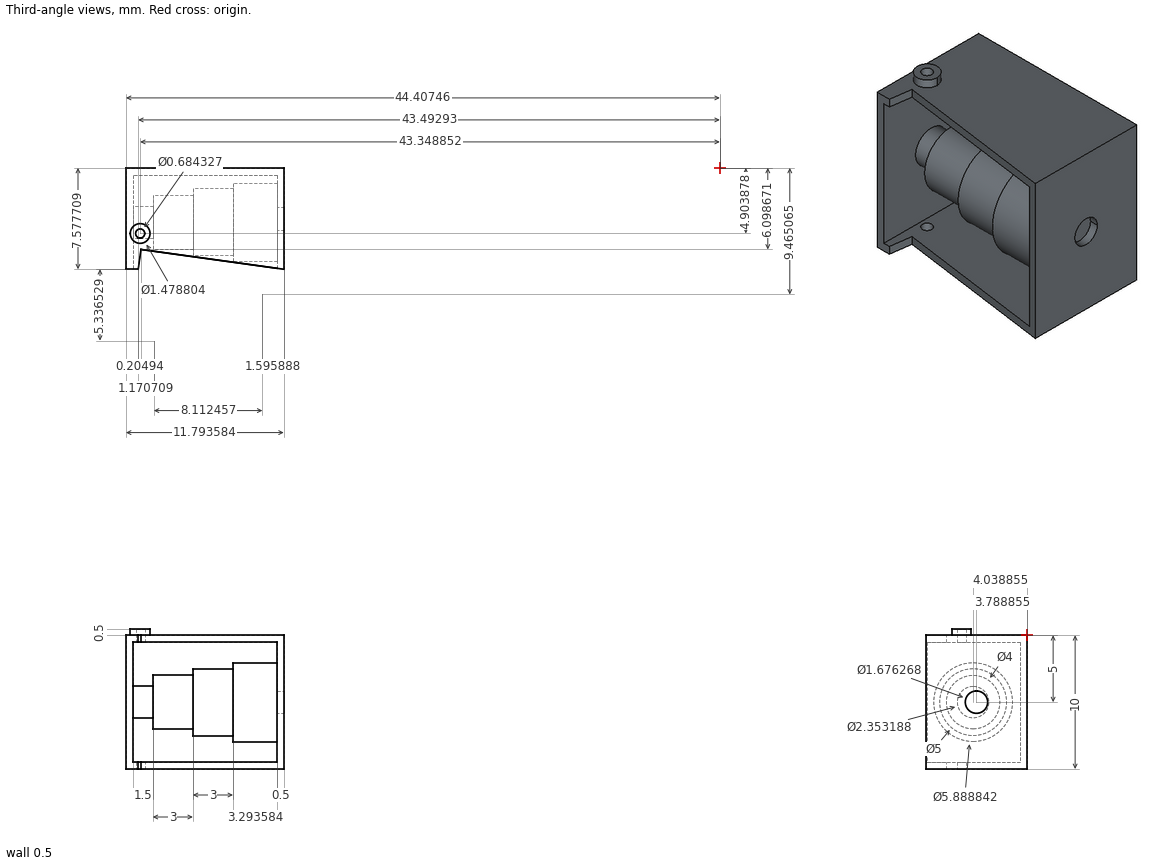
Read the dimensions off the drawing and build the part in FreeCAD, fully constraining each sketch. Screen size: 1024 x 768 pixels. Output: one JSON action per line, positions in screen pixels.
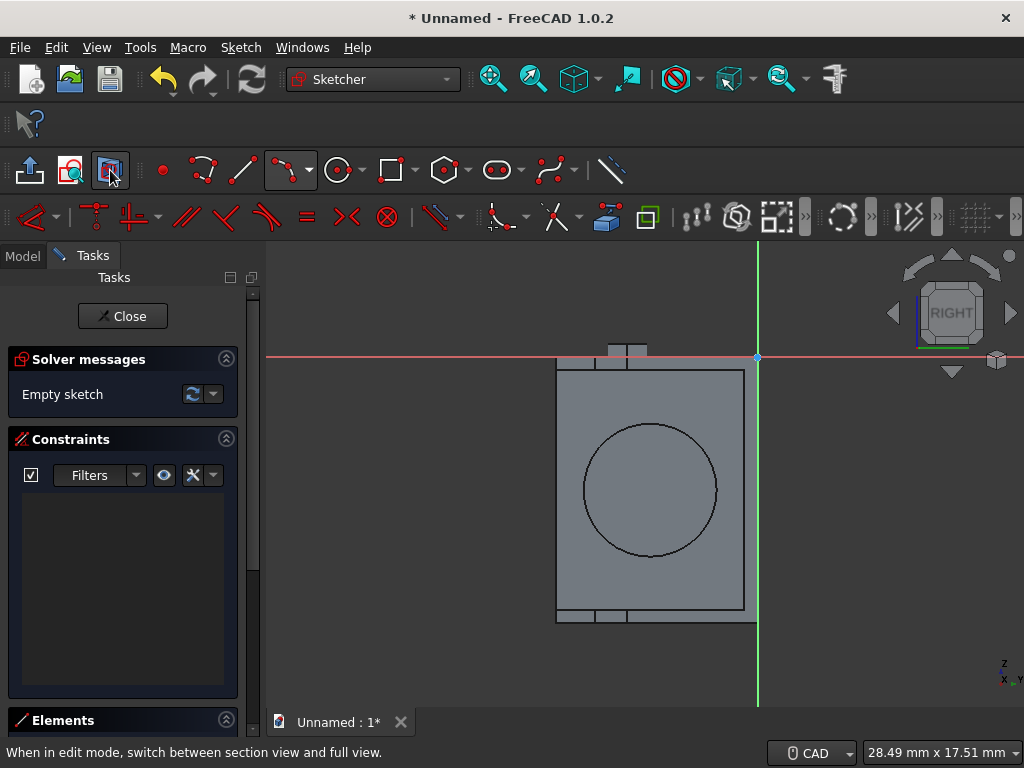
{"action": "scroll", "coordinate": [844, 440], "scroll_direction": "up", "scroll_amount": 2}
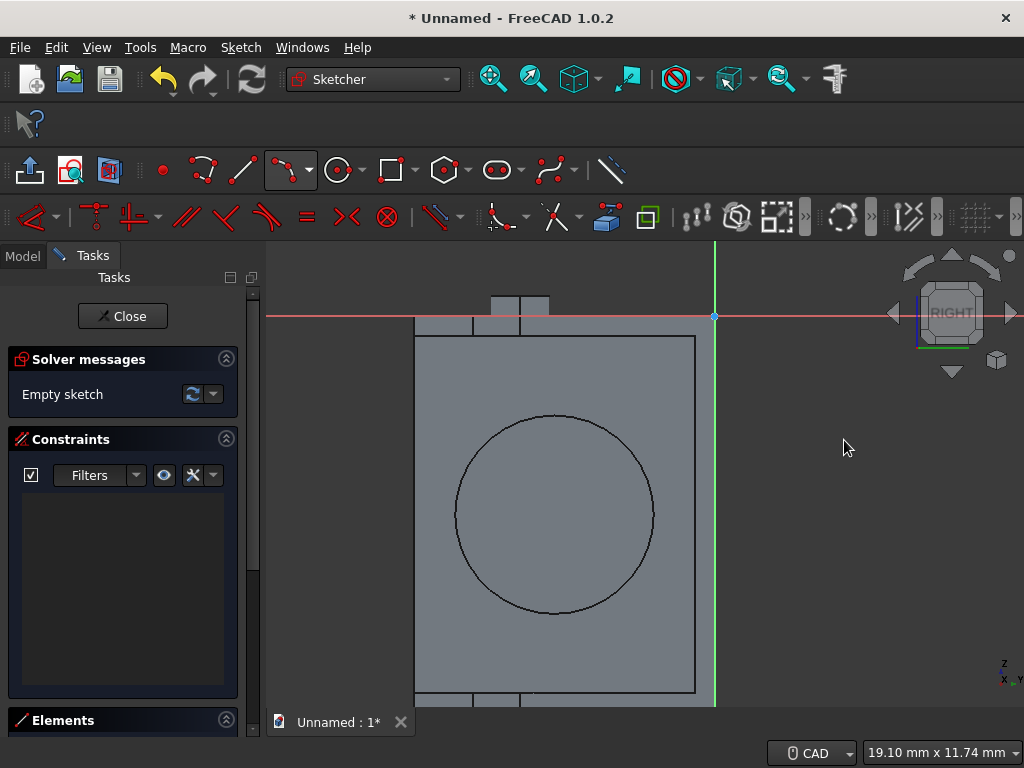
{"action": "left_click", "coordinate": [338, 170]}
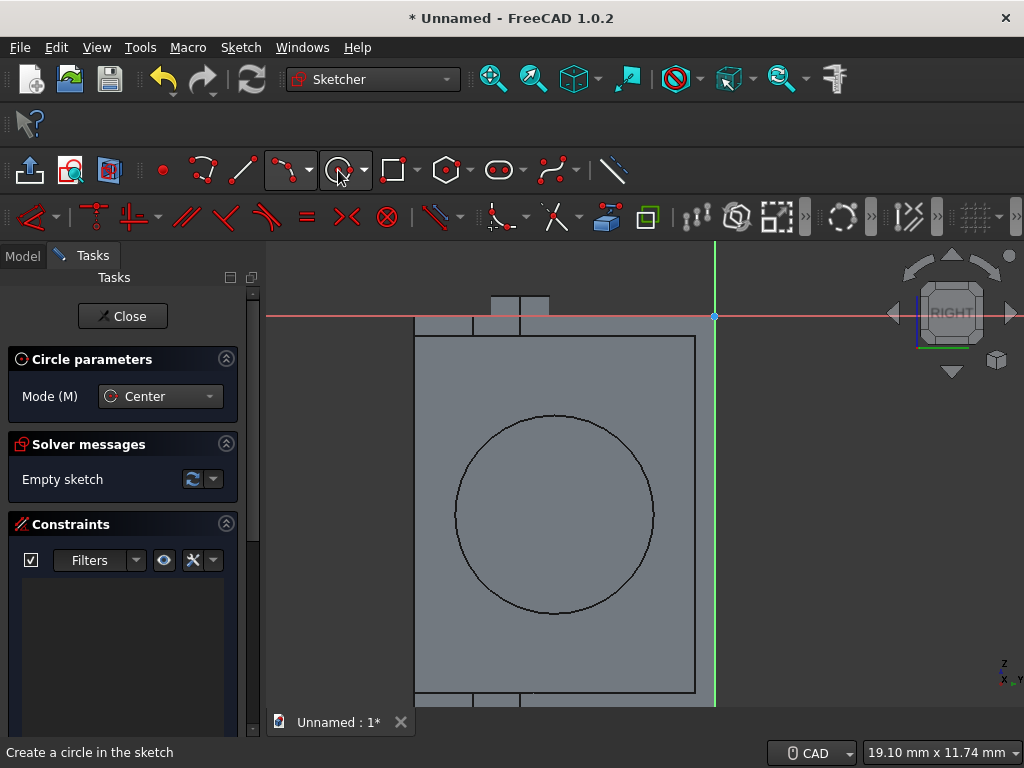
{"action": "left_click", "coordinate": [554, 515]}
{"action": "left_click", "coordinate": [637, 432]}
{"action": "key", "text": "Escape"}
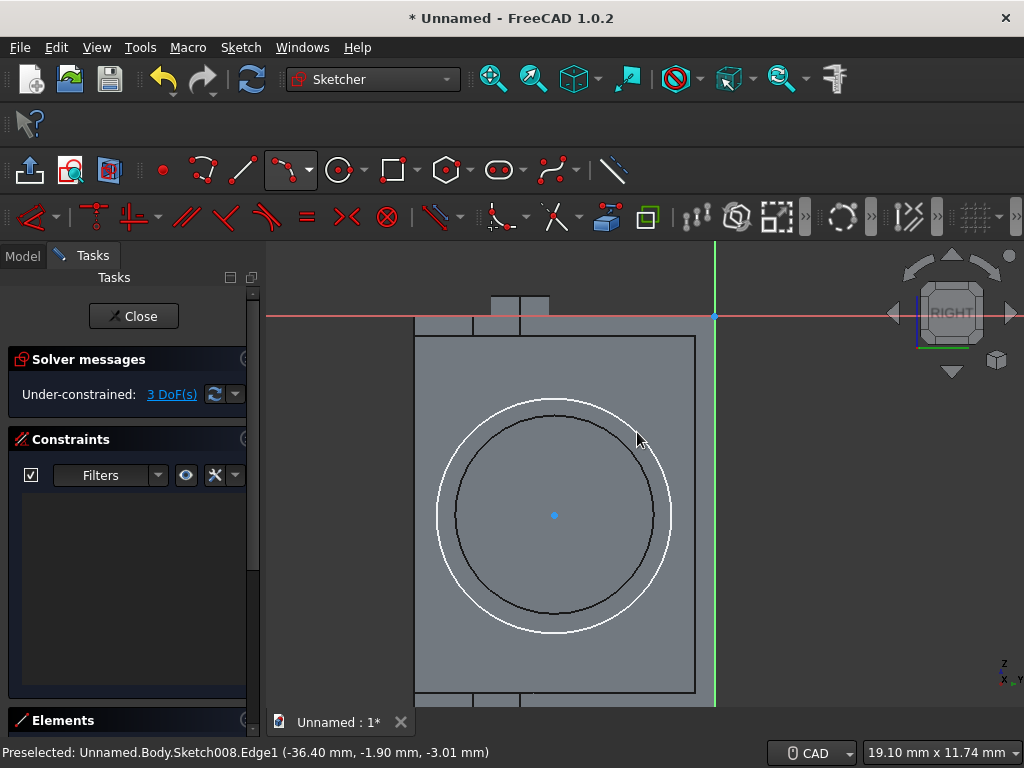
{"action": "left_click", "coordinate": [32, 218]}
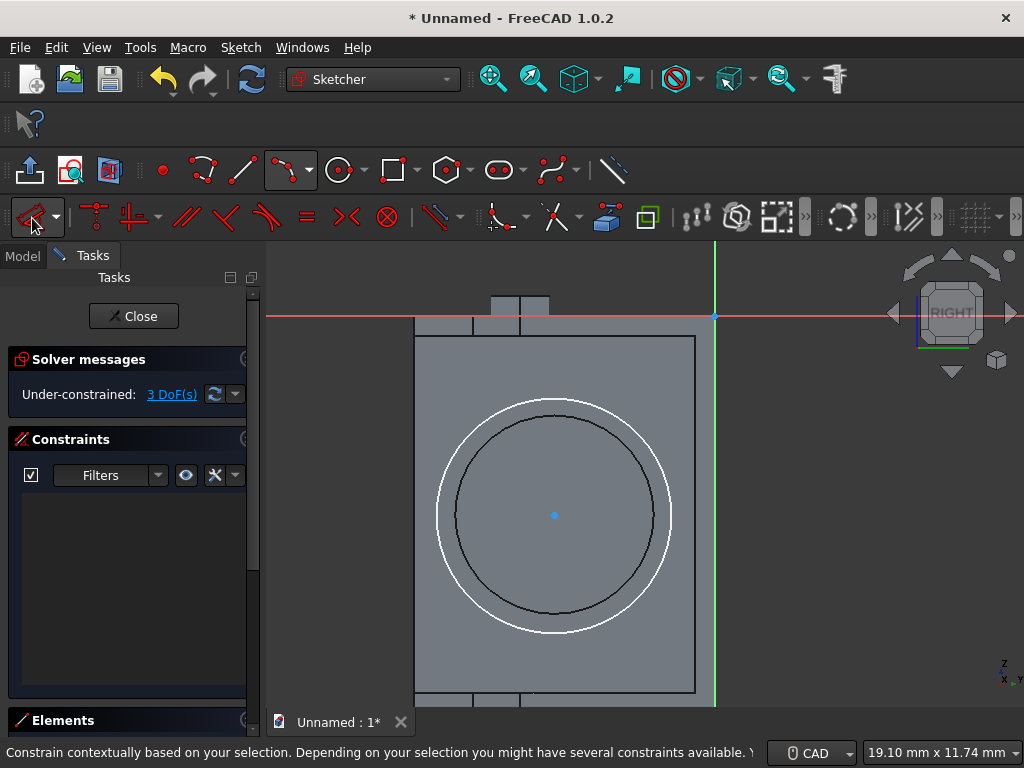
{"action": "left_click", "coordinate": [637, 433]}
{"action": "left_click", "coordinate": [660, 410]}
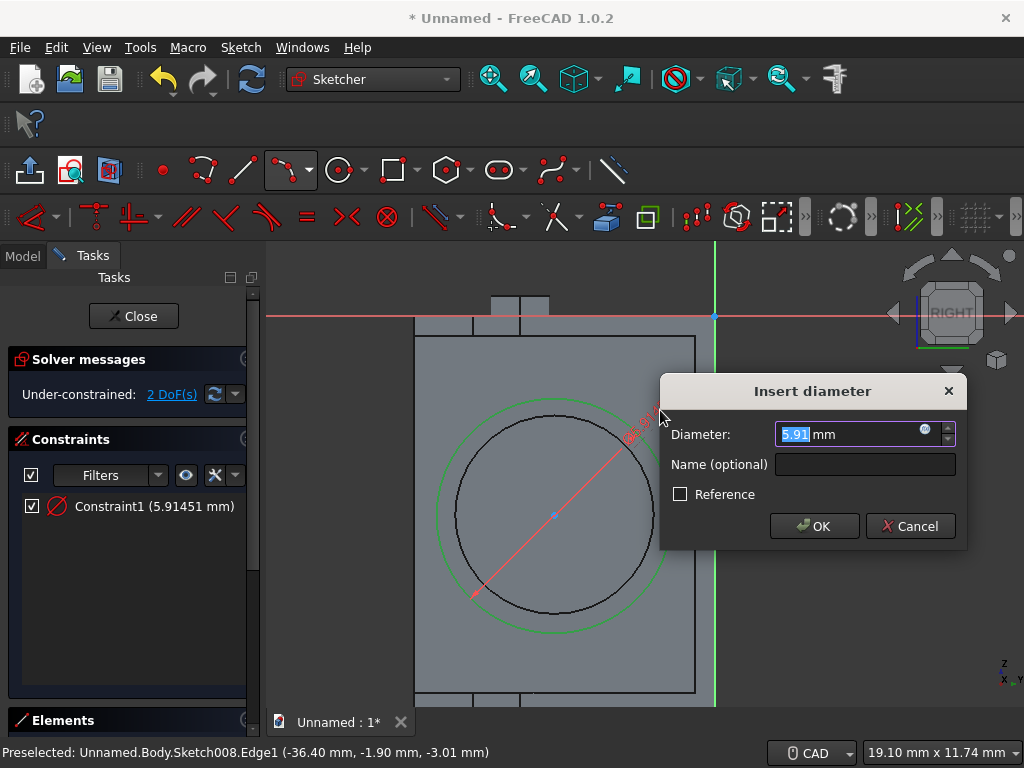
{"action": "type", "text": "5.888842"}
{"action": "key", "text": "Return"}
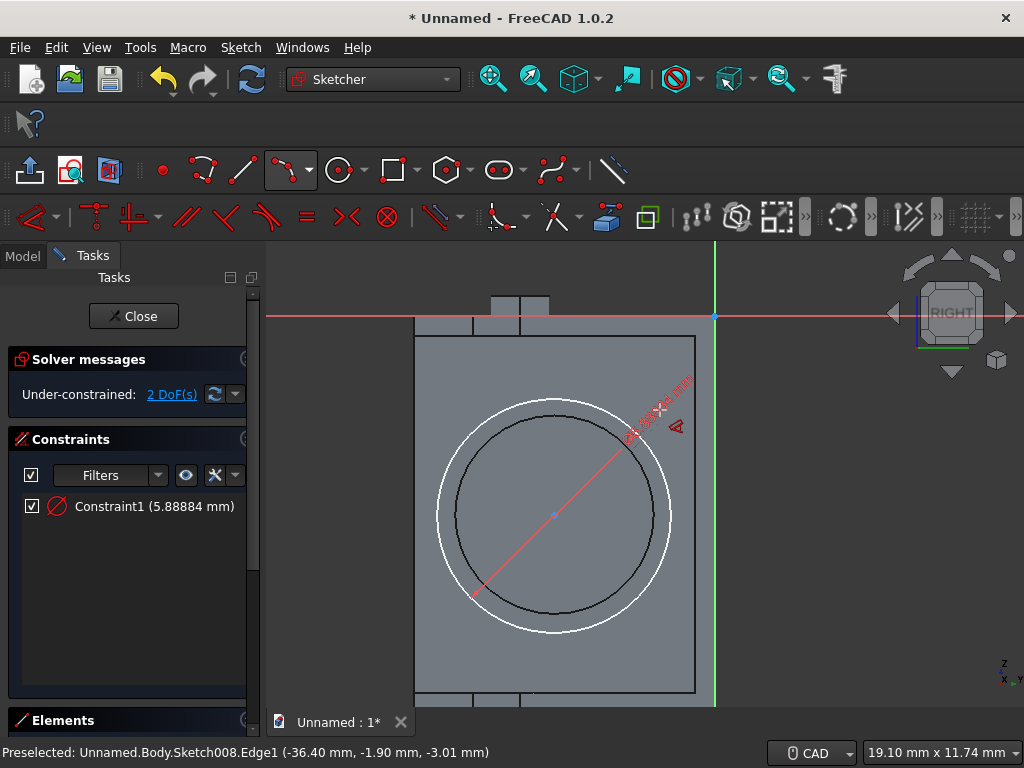
{"action": "left_click", "coordinate": [554, 516]}
{"action": "left_click", "coordinate": [749, 416]}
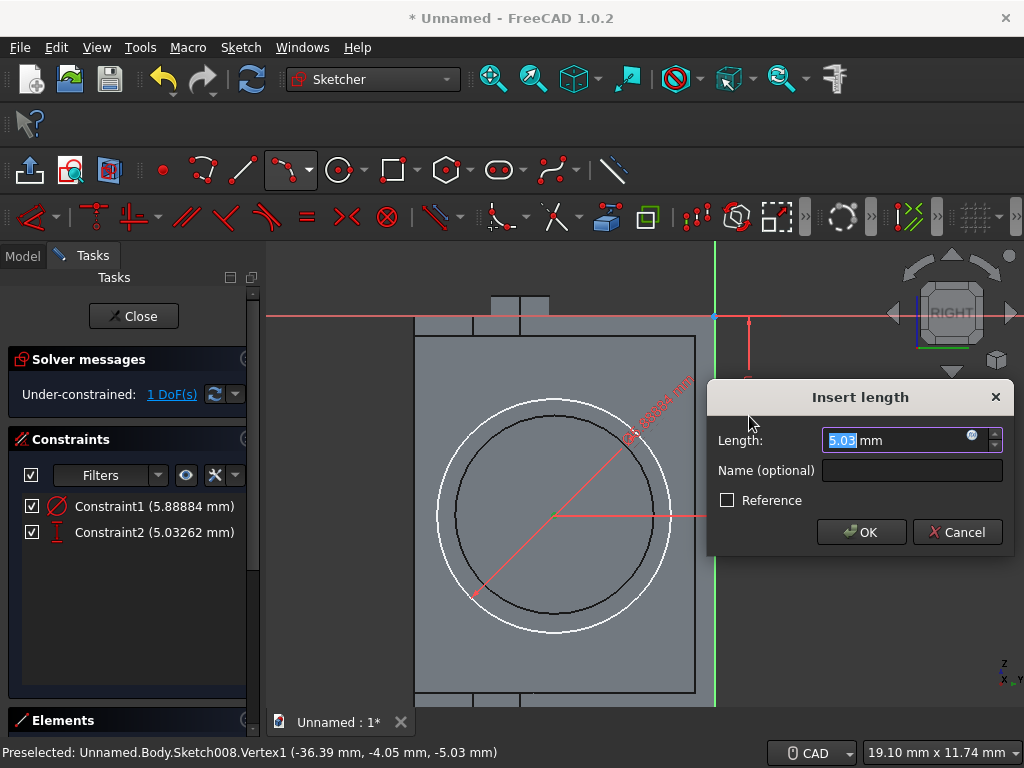
{"action": "type", "text": "5"}
{"action": "key", "text": "Return"}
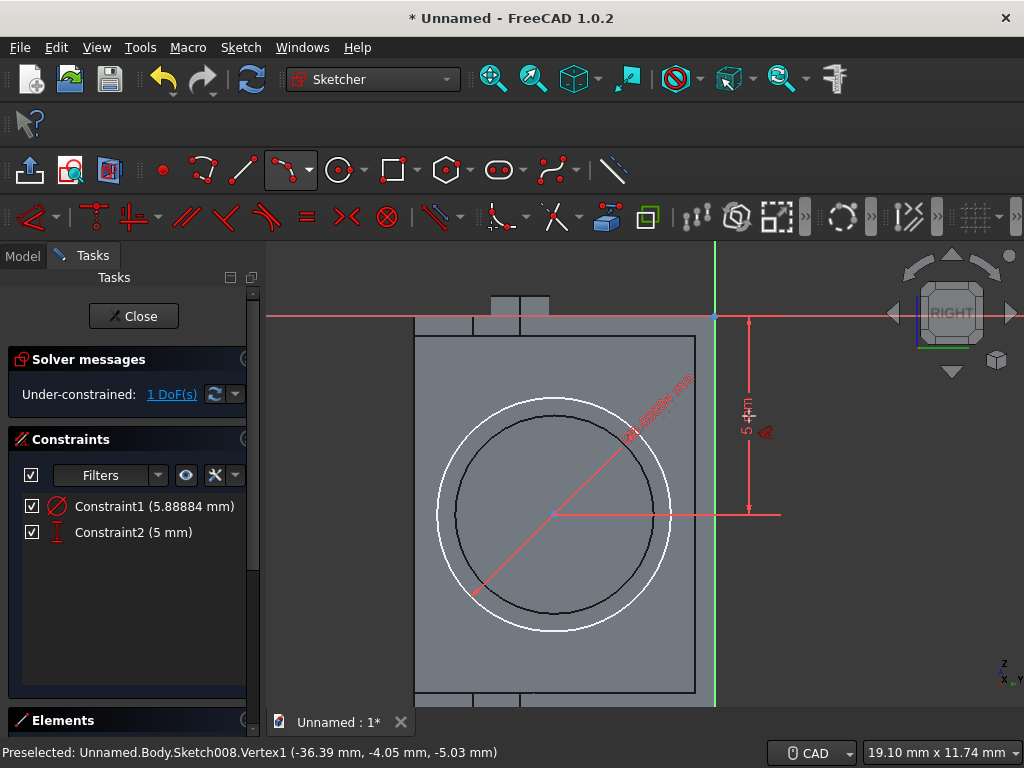
{"action": "left_click", "coordinate": [554, 515]}
{"action": "left_click", "coordinate": [634, 282]}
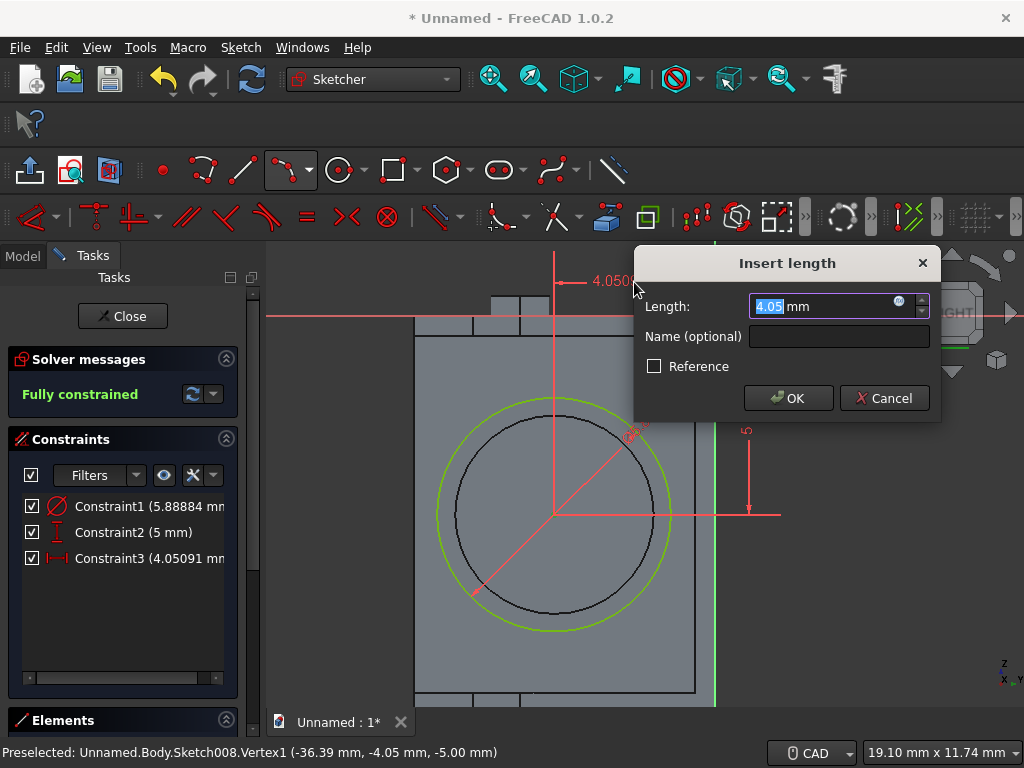
{"action": "type", "text": "4.038855"}
{"action": "key", "text": "Return"}
{"action": "key", "text": "Escape"}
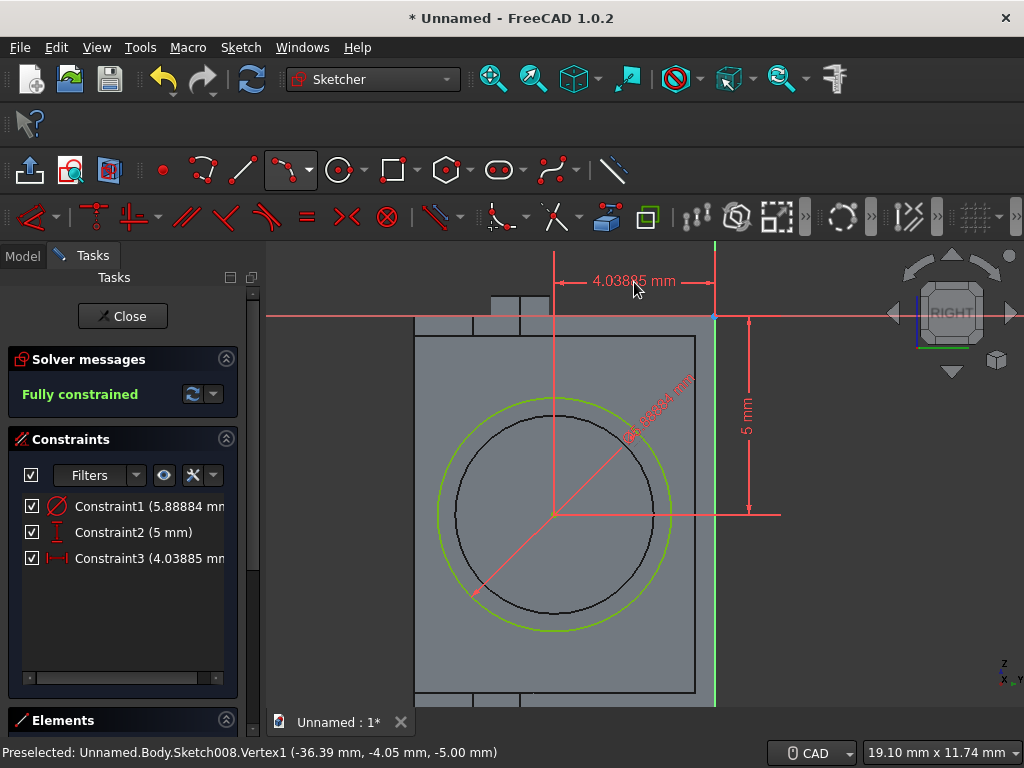
{"action": "left_click", "coordinate": [123, 316]}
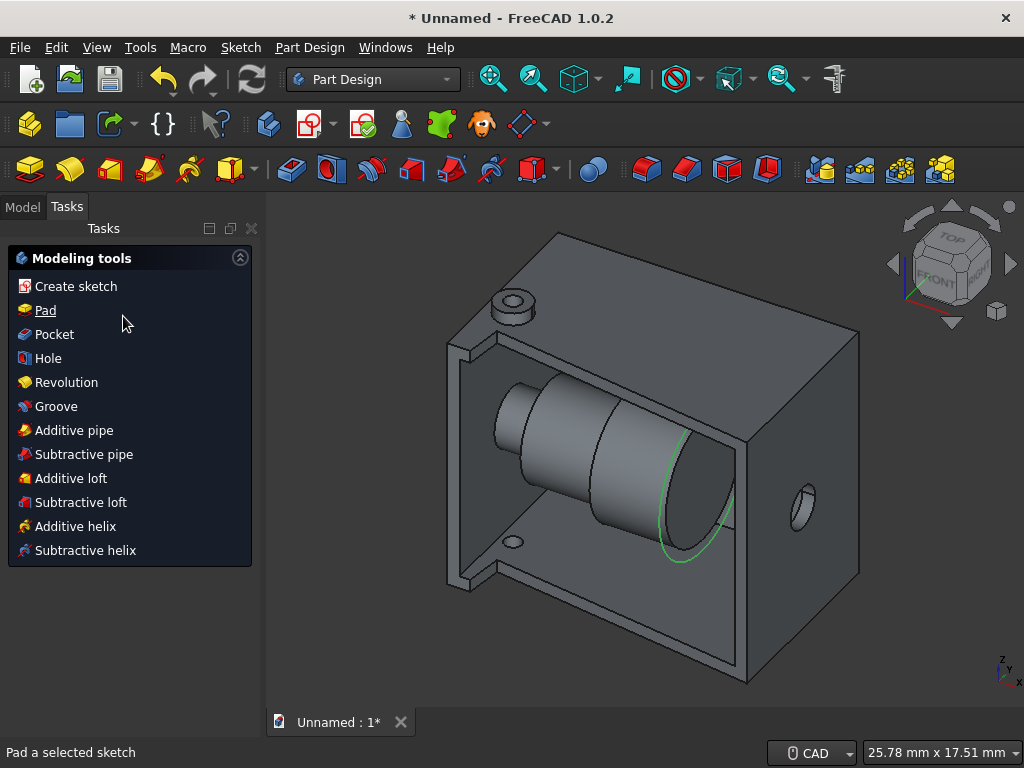
{"action": "left_click", "coordinate": [30, 170]}